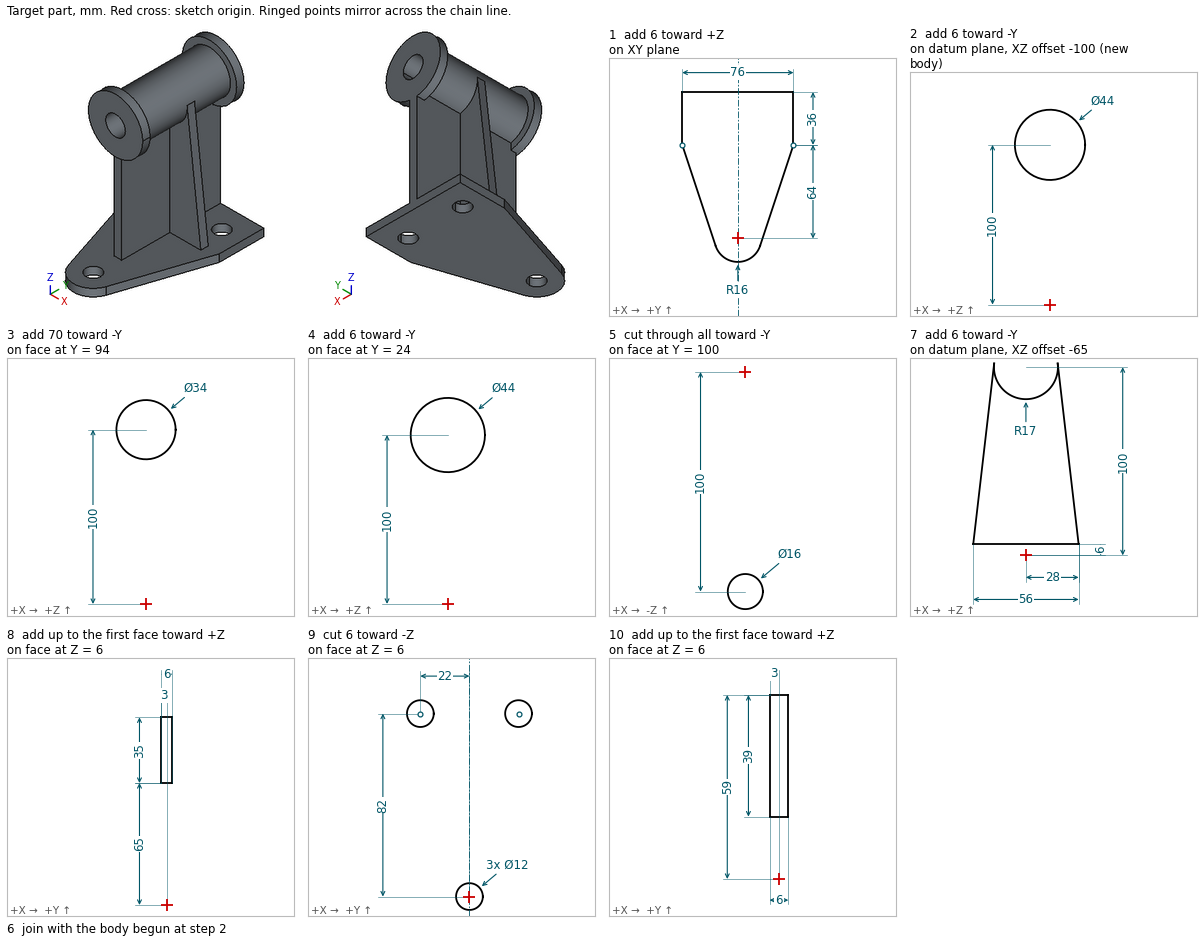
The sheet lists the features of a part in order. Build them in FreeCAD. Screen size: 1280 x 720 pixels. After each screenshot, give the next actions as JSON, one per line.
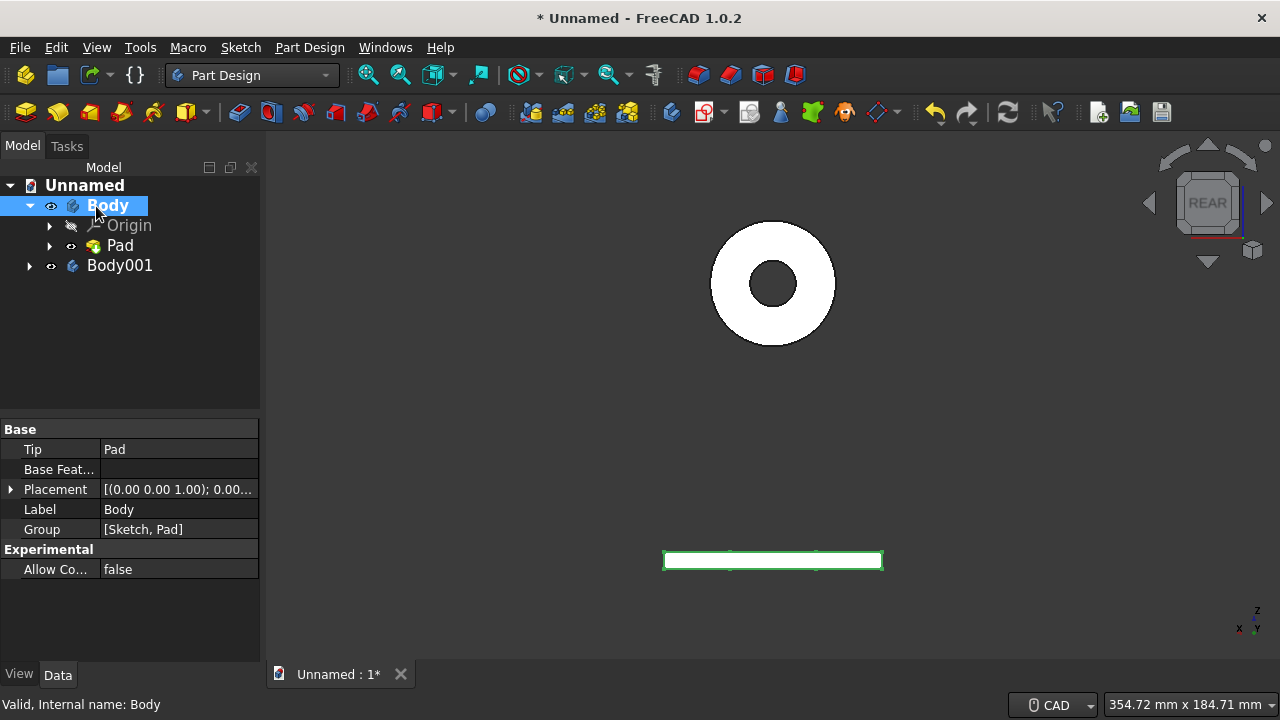
{"action": "left_click", "coordinate": [146, 569]}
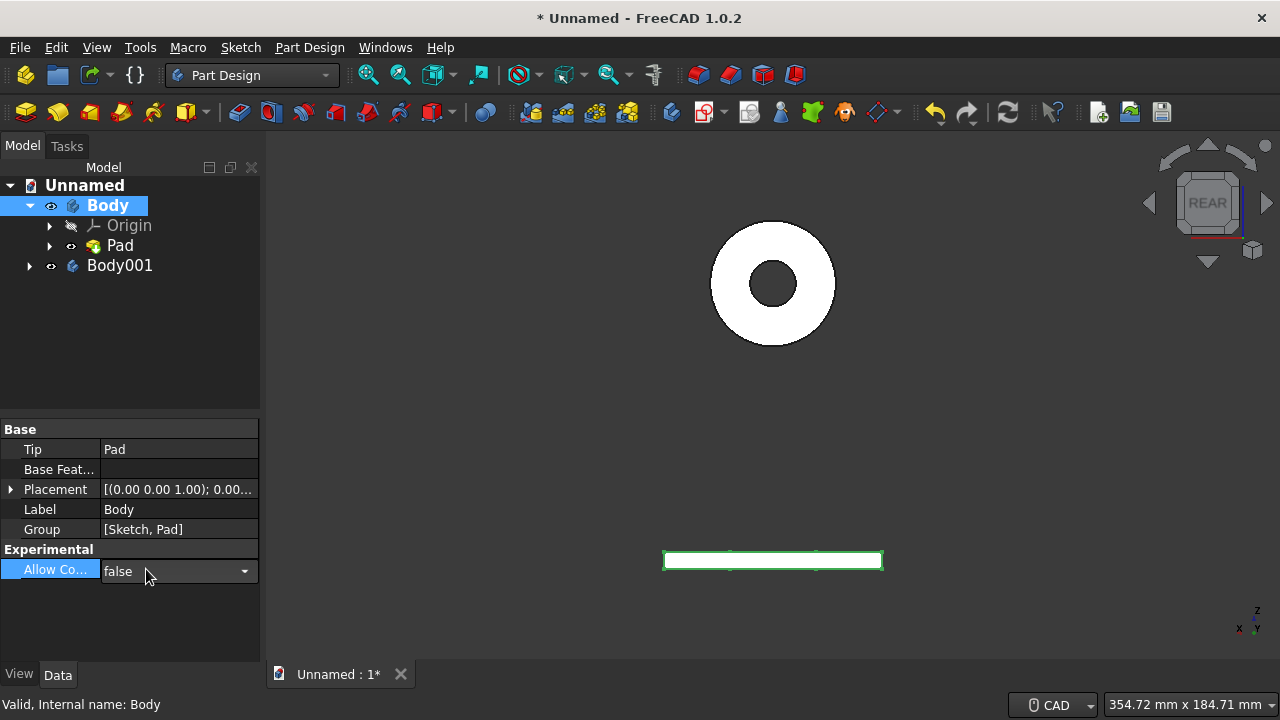
{"action": "left_click", "coordinate": [146, 569]}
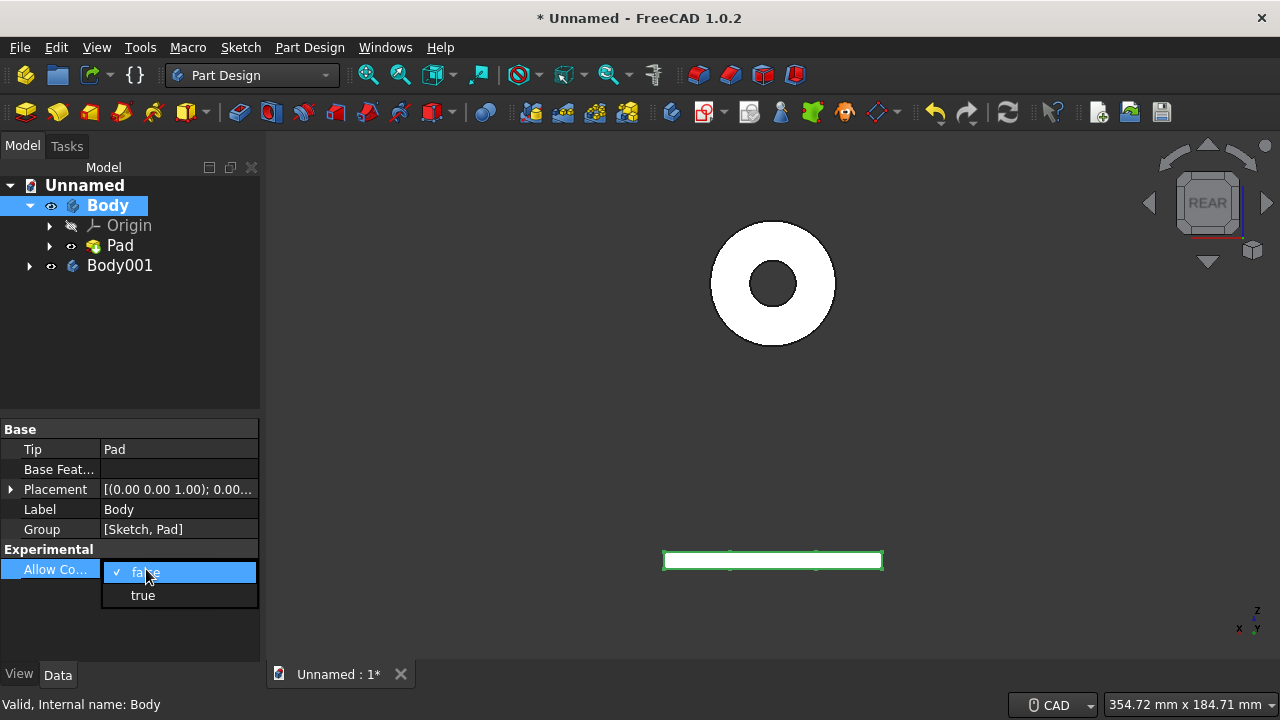
{"action": "left_click", "coordinate": [179, 596]}
{"action": "key", "text": "Return"}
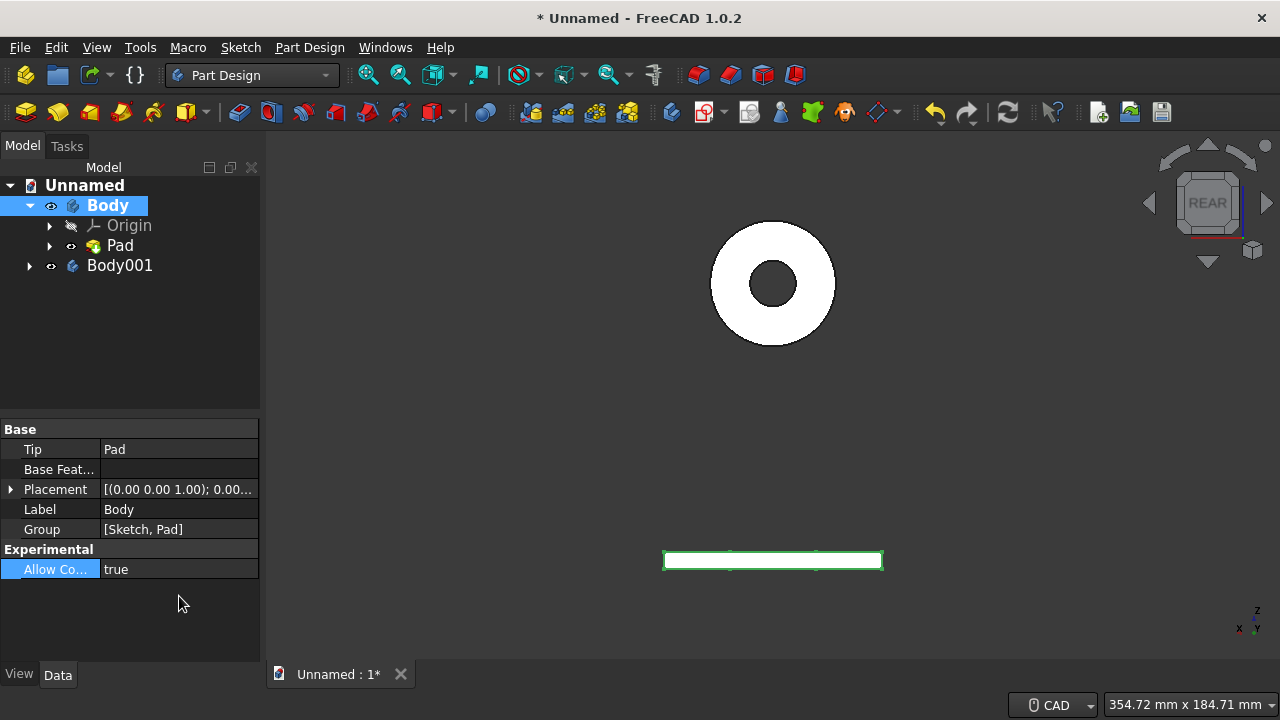
{"action": "left_click", "coordinate": [96, 266]}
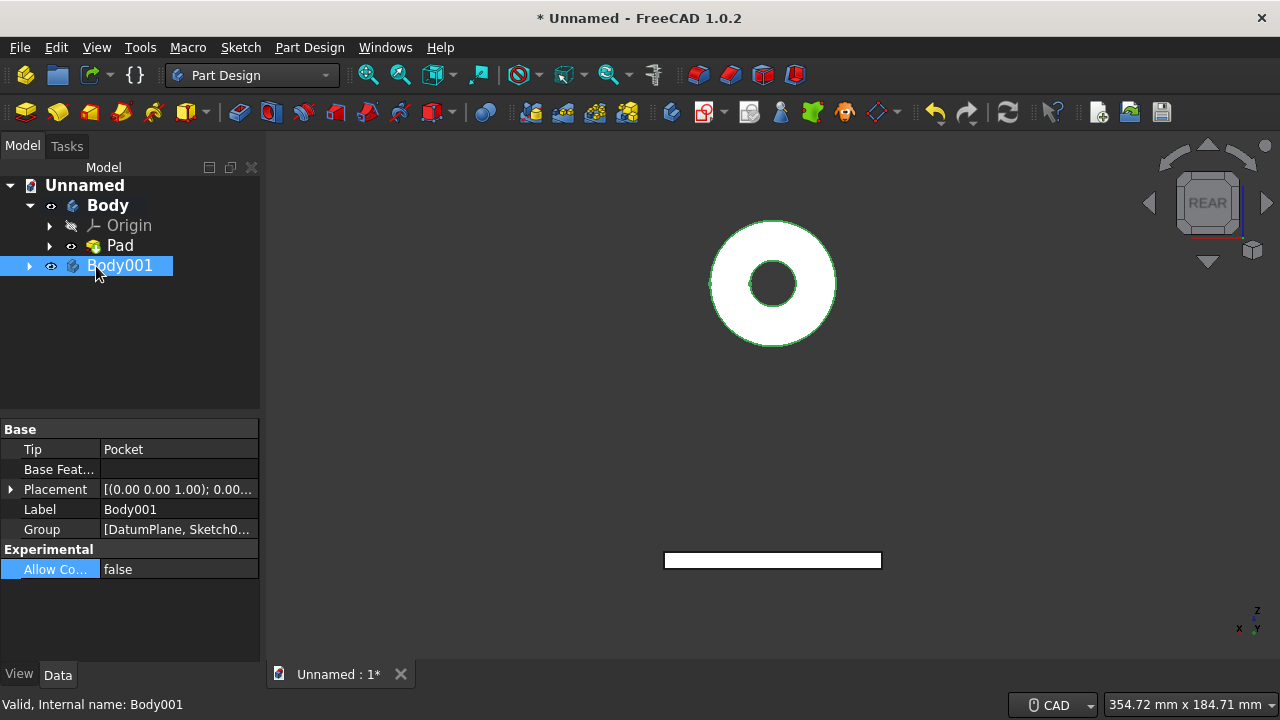
{"action": "left_click", "coordinate": [486, 112]}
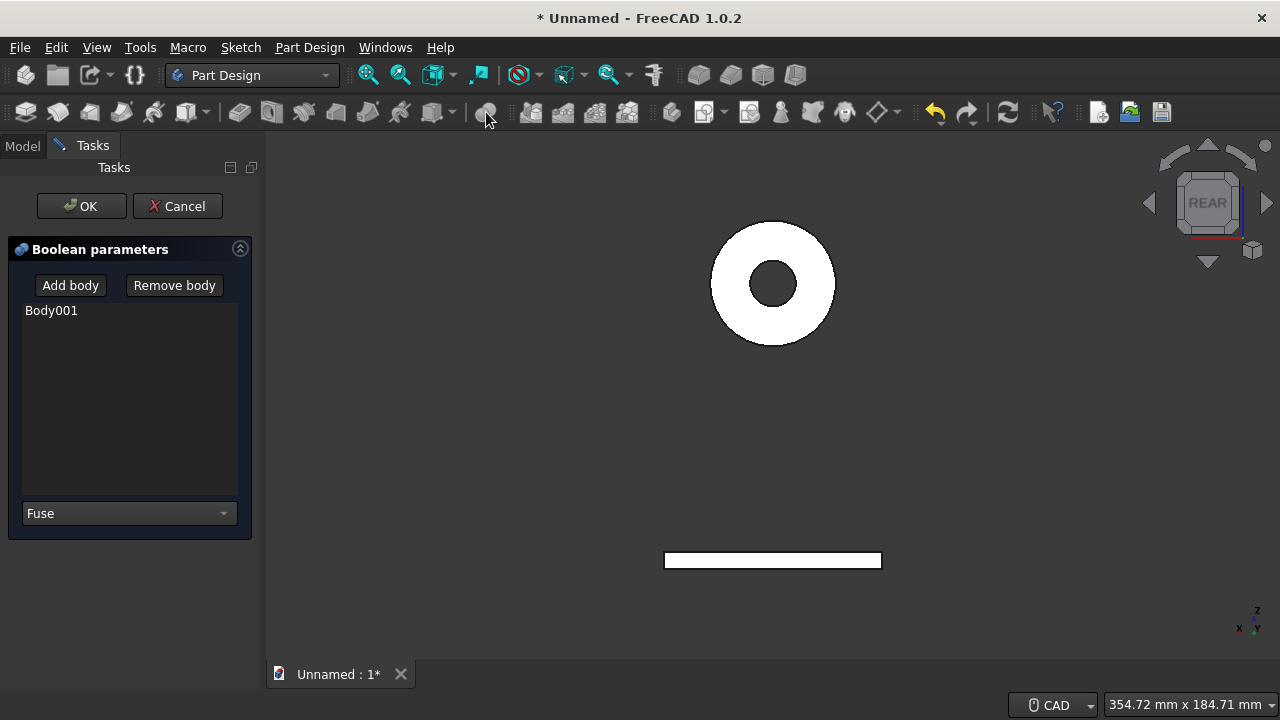
{"action": "left_click", "coordinate": [82, 206]}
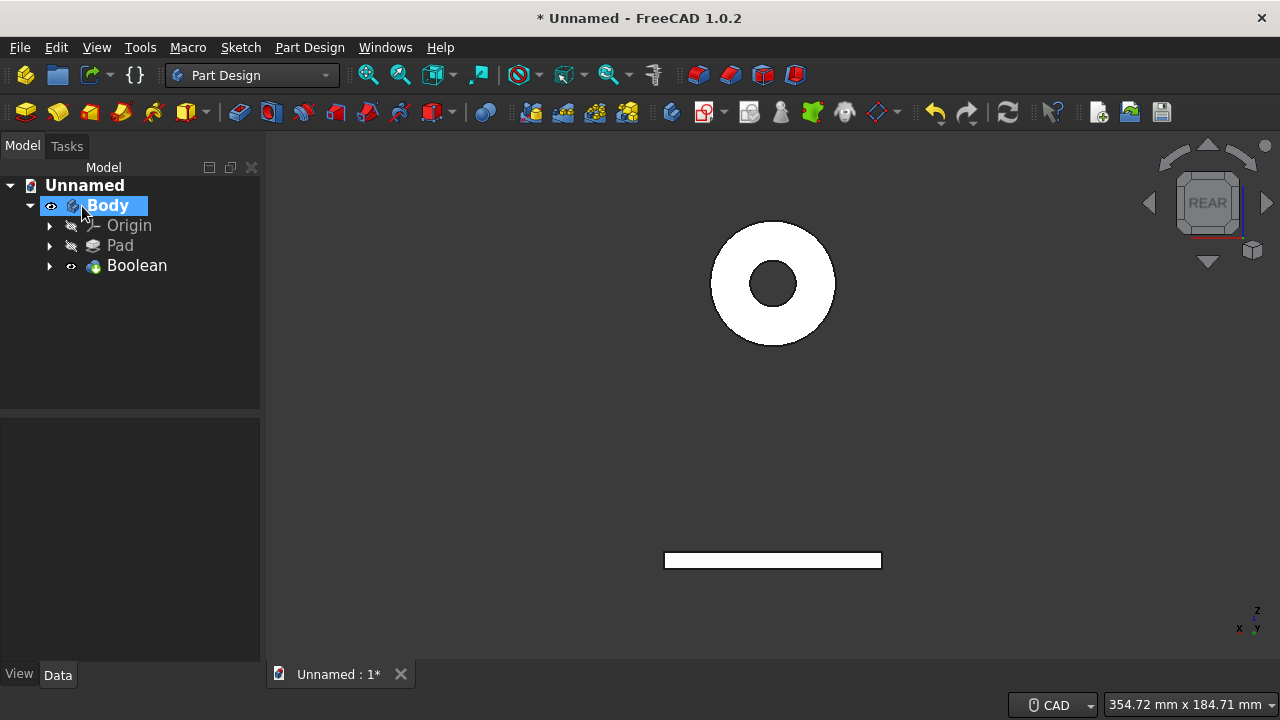
{"action": "left_click", "coordinate": [50, 226]}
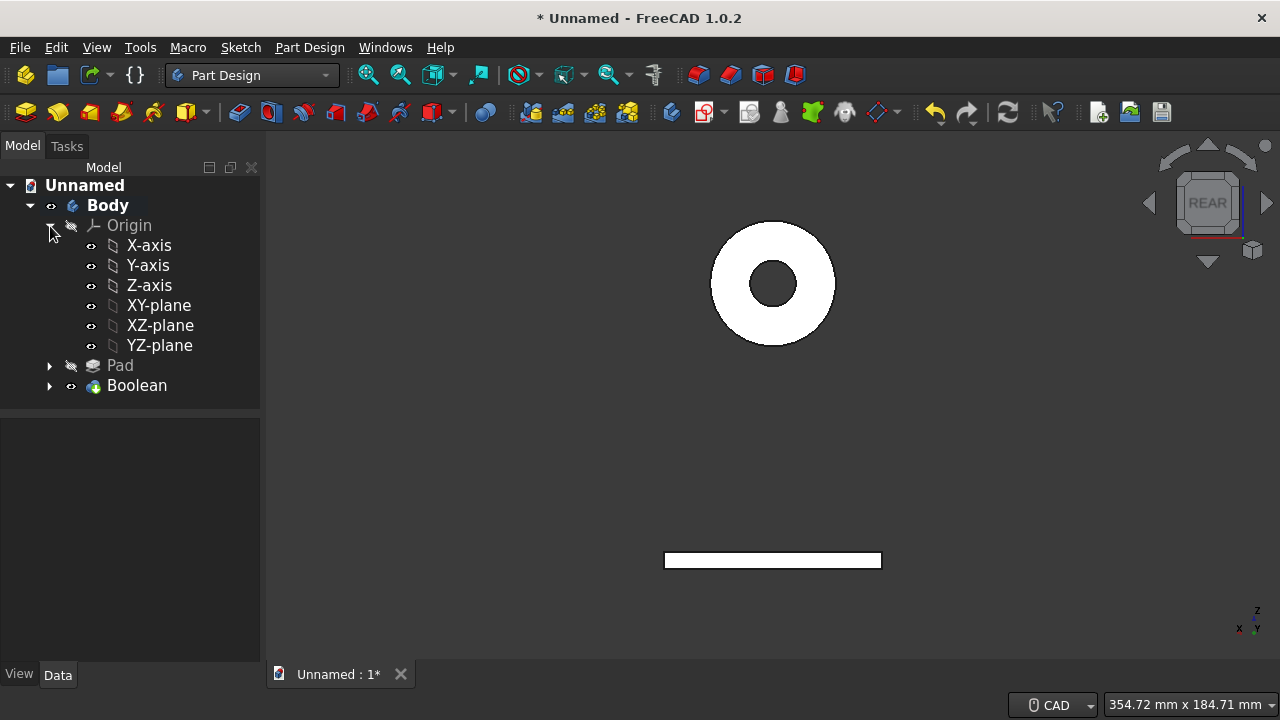
{"action": "left_click", "coordinate": [136, 326]}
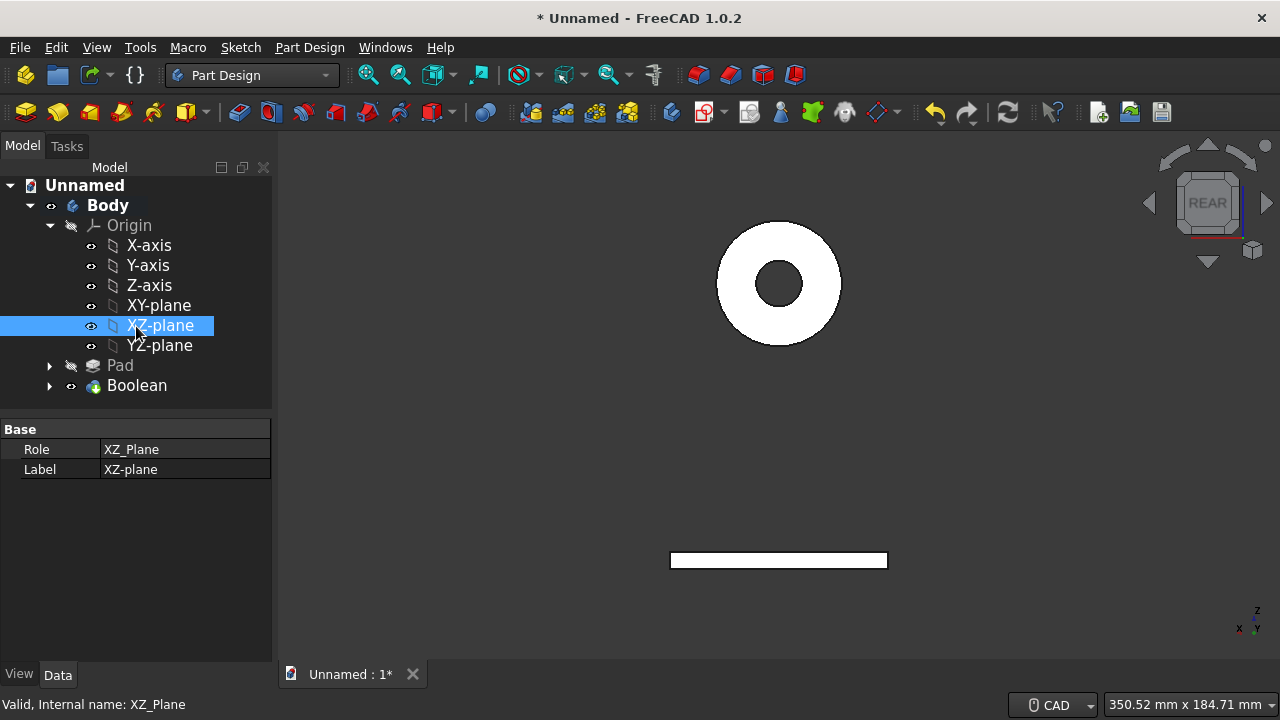
{"action": "left_click", "coordinate": [878, 112]}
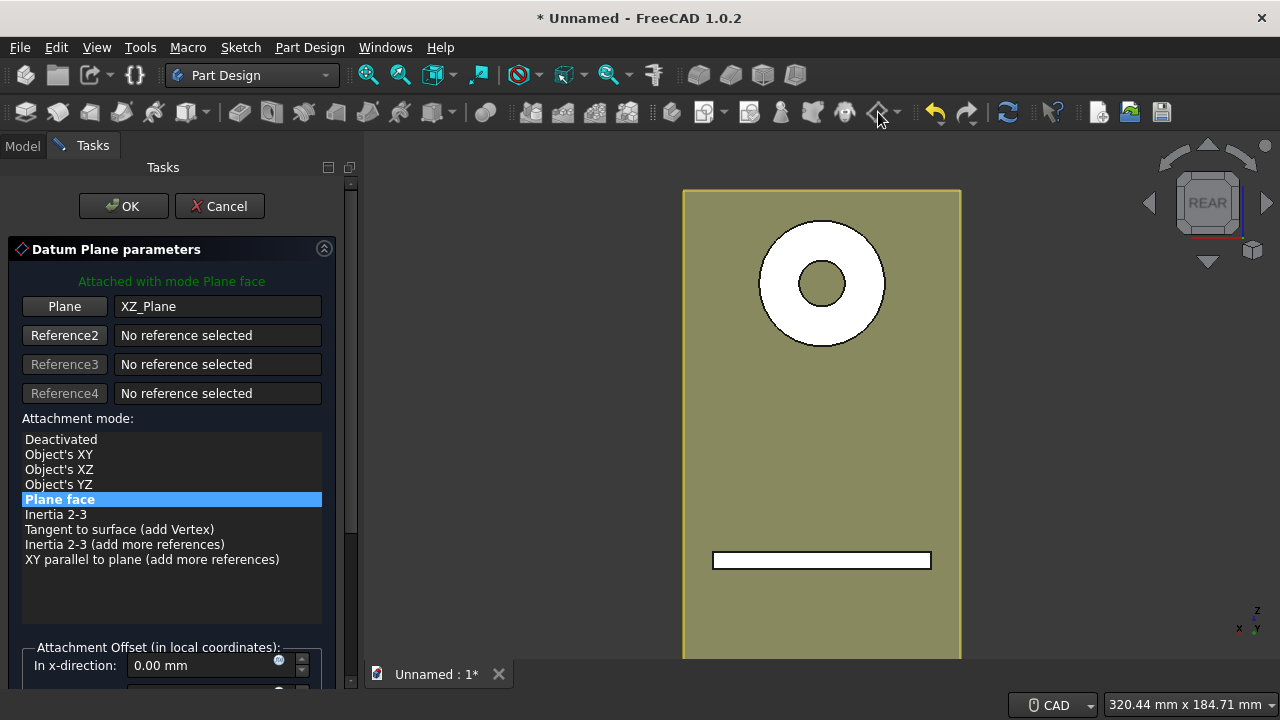
{"action": "scroll", "coordinate": [351, 432], "scroll_direction": "down", "scroll_amount": 2}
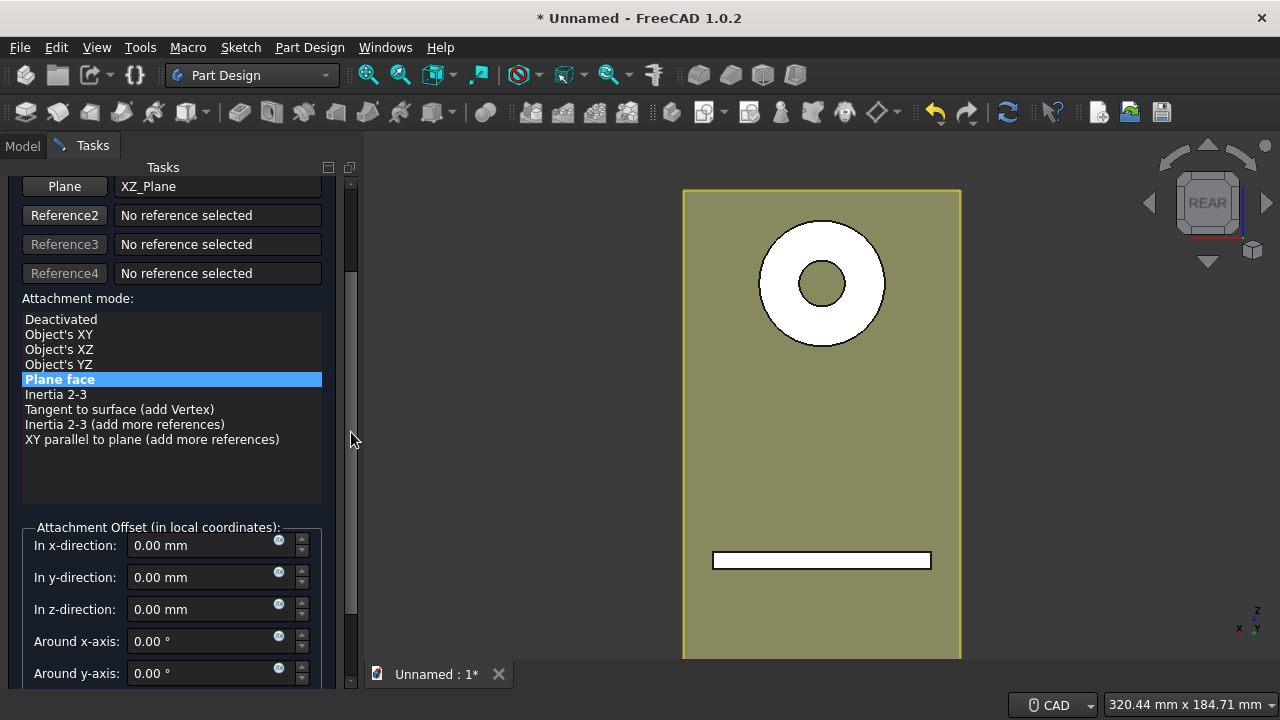
{"action": "triple_click", "coordinate": [210, 609]}